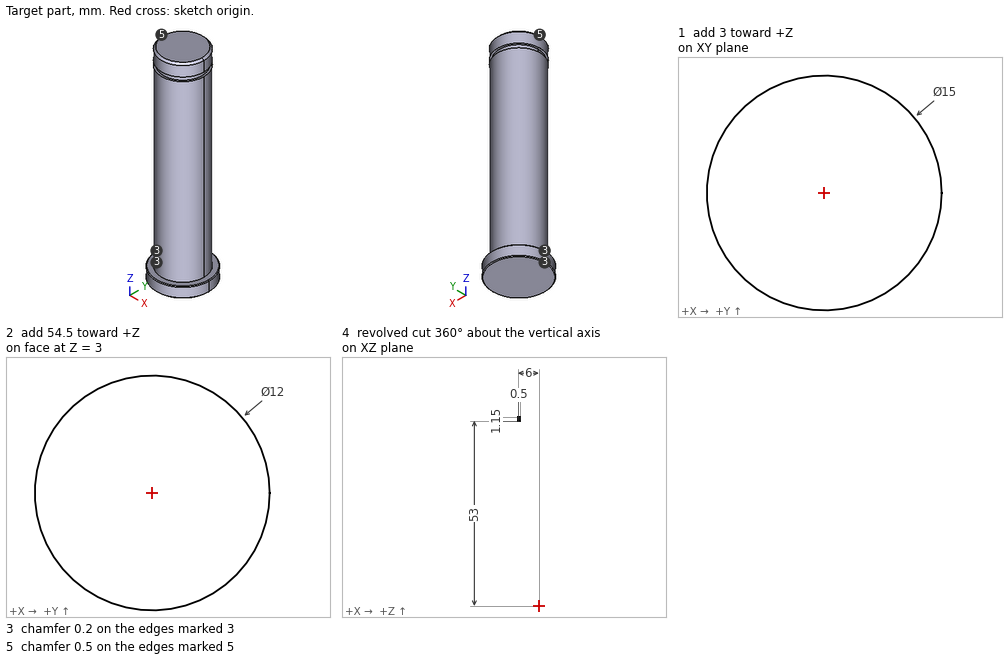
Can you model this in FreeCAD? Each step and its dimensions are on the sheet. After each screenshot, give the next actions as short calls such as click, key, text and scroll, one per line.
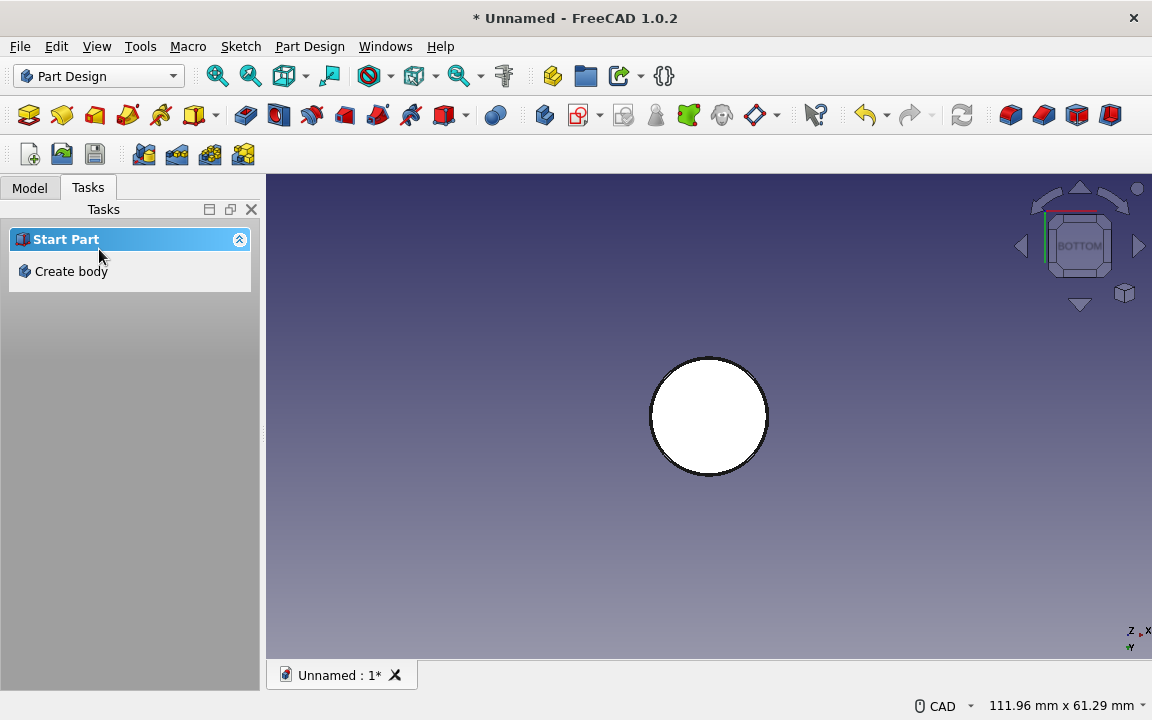
click(578, 116)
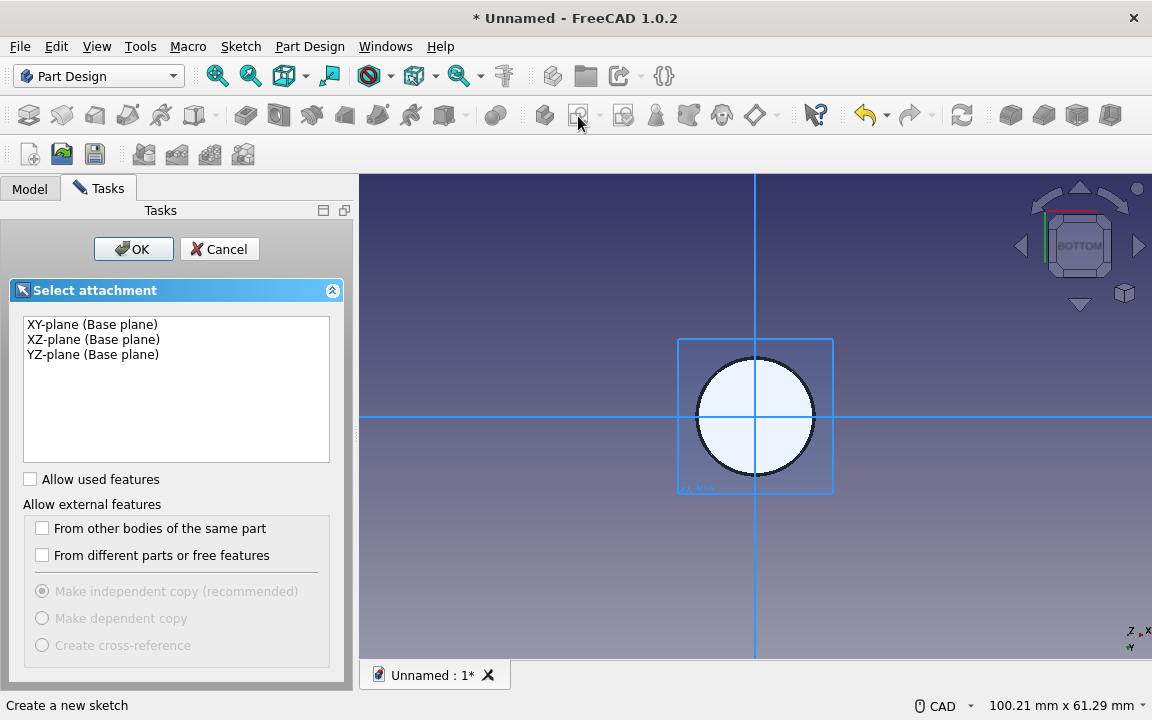
click(84, 340)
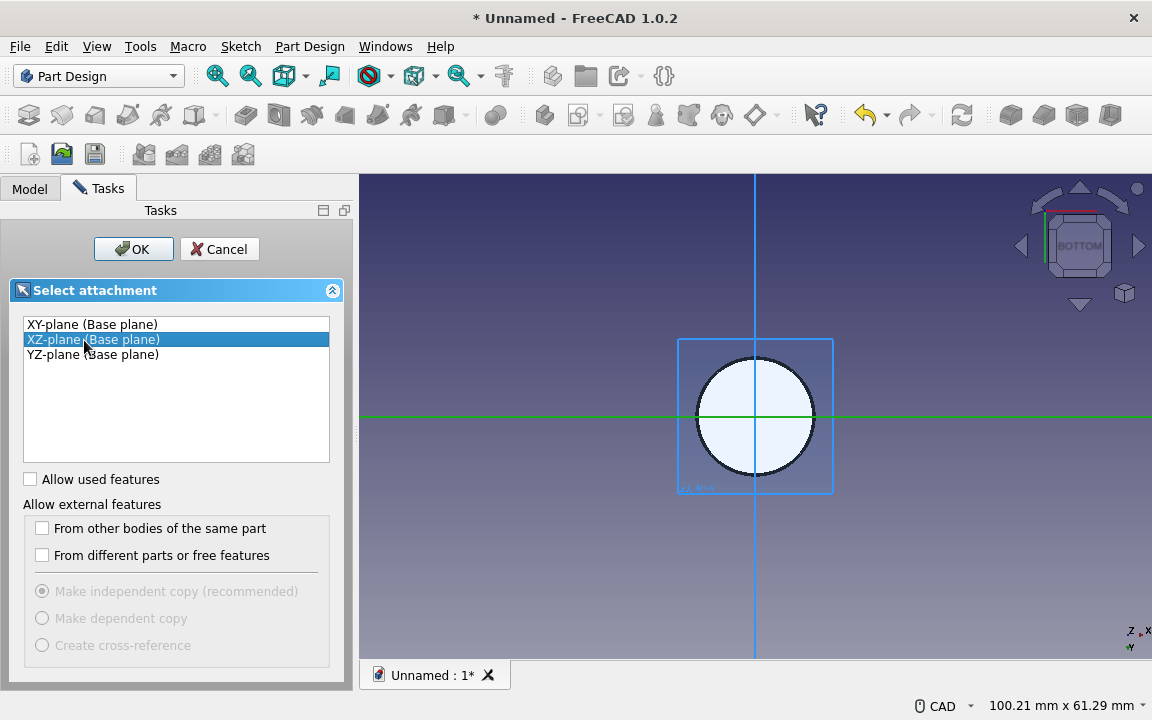
click(134, 249)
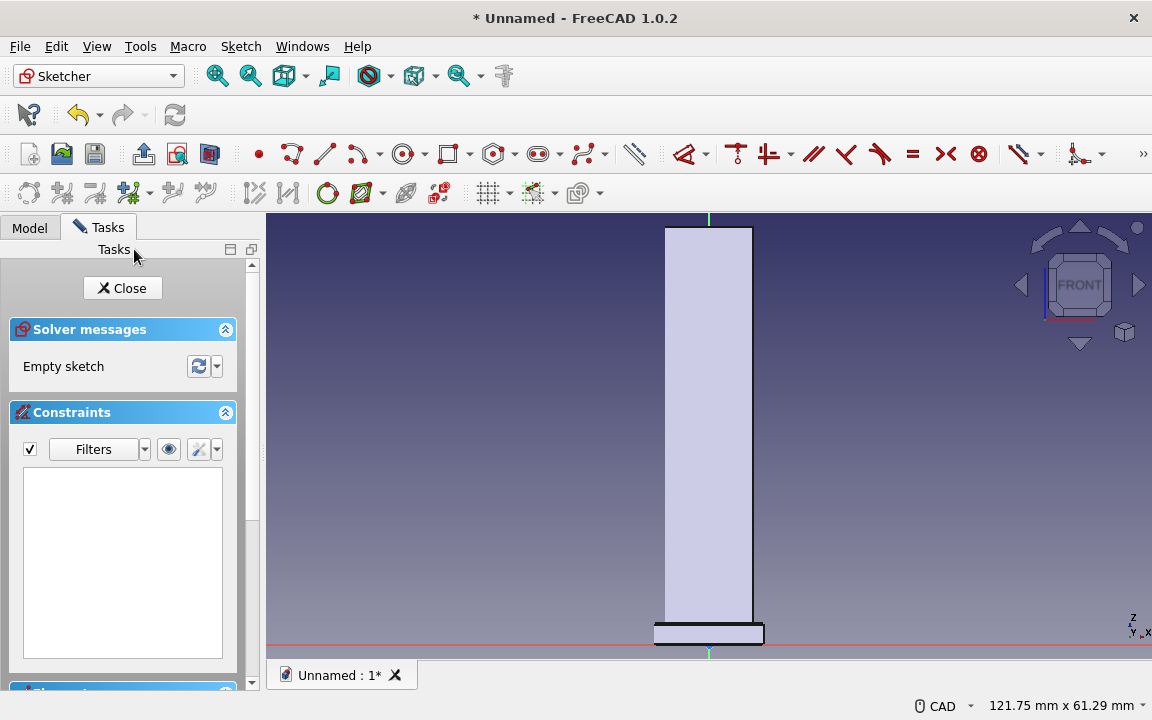
key(q)
key(s)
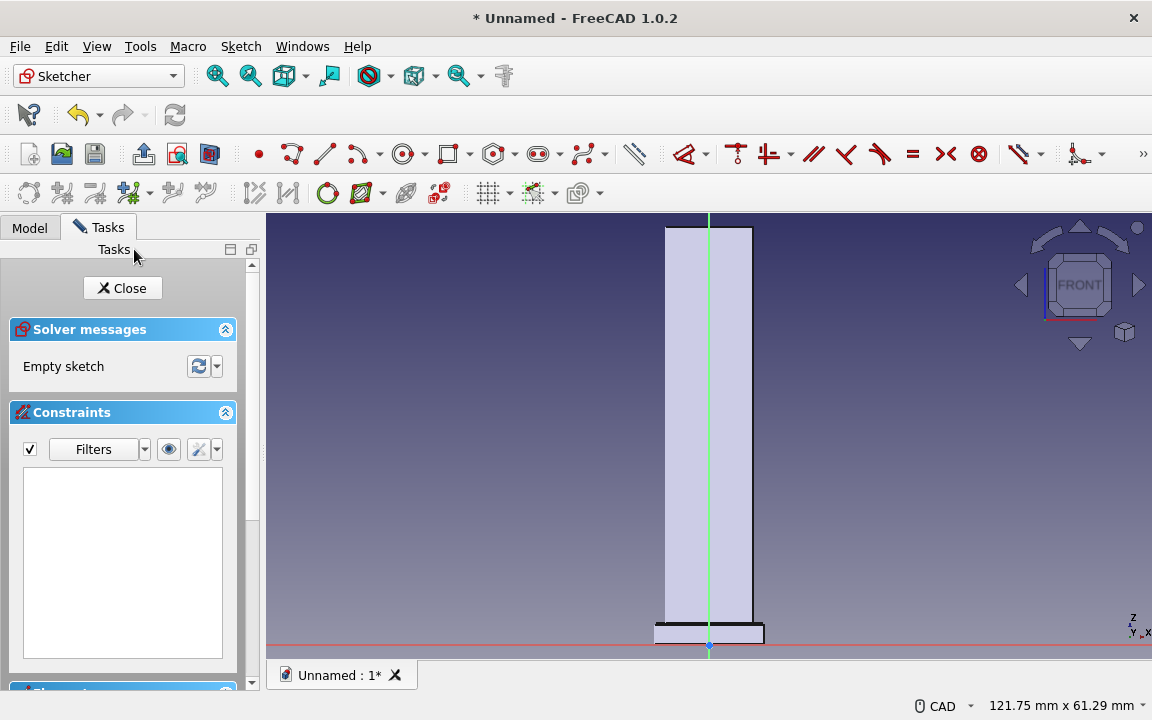
scroll(669, 246, up, 15)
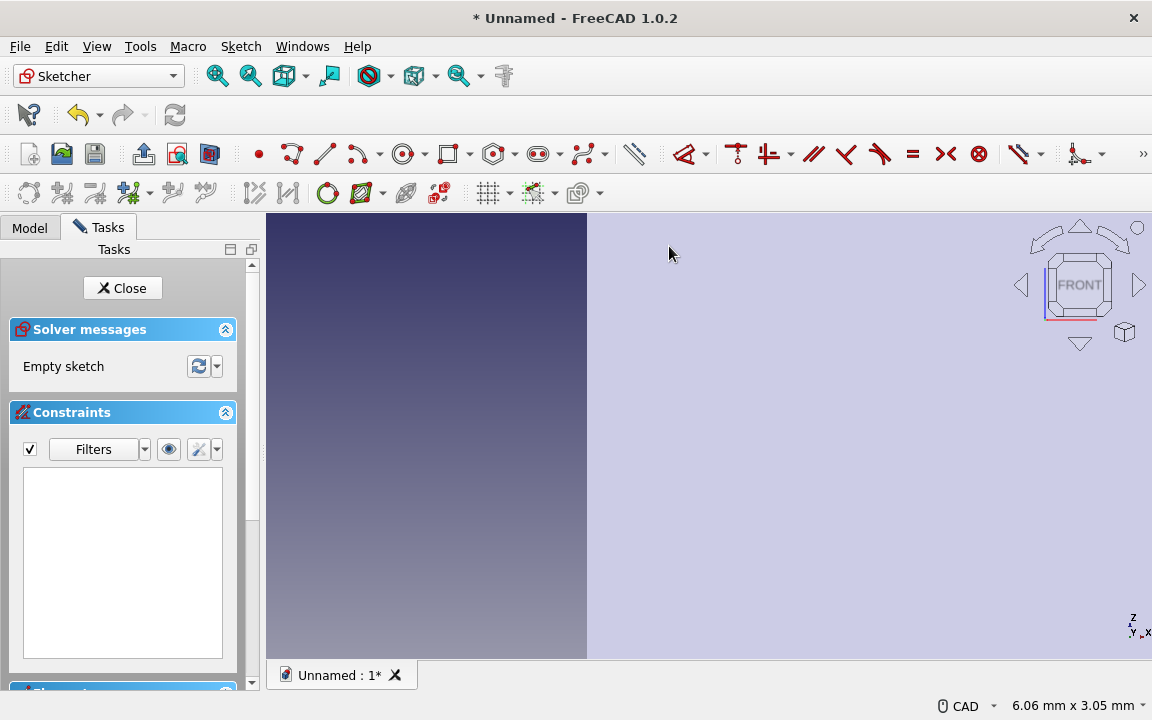
scroll(588, 425, up, 2)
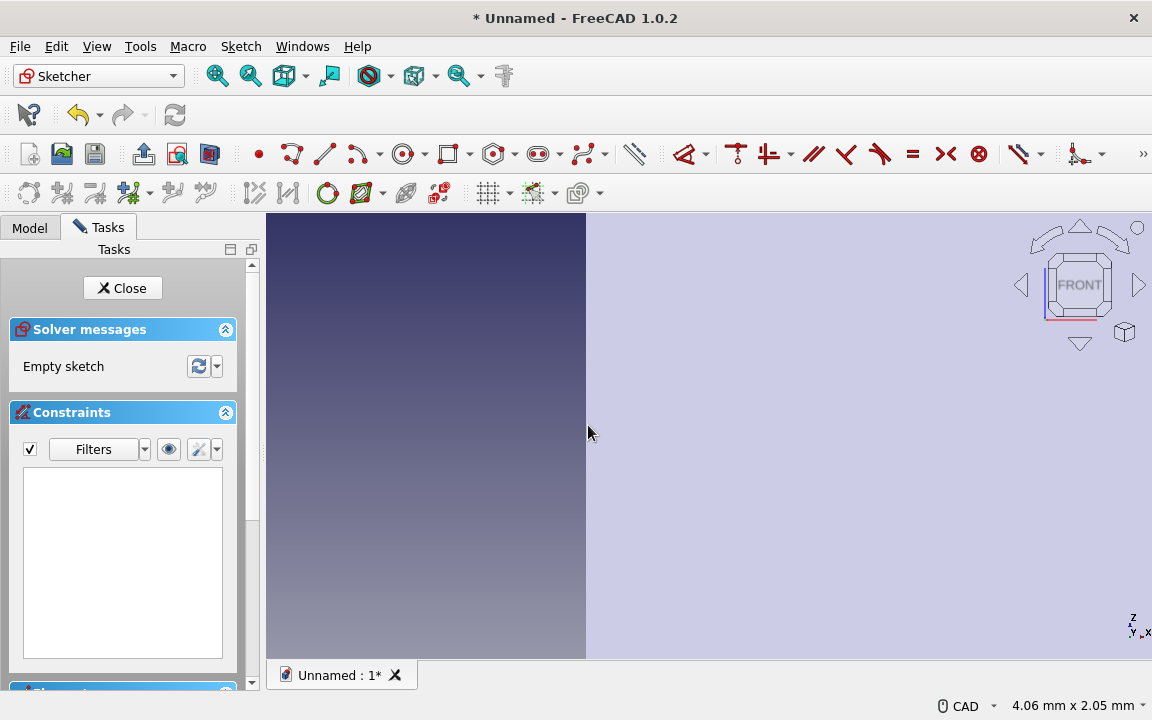
key(g)
key(r)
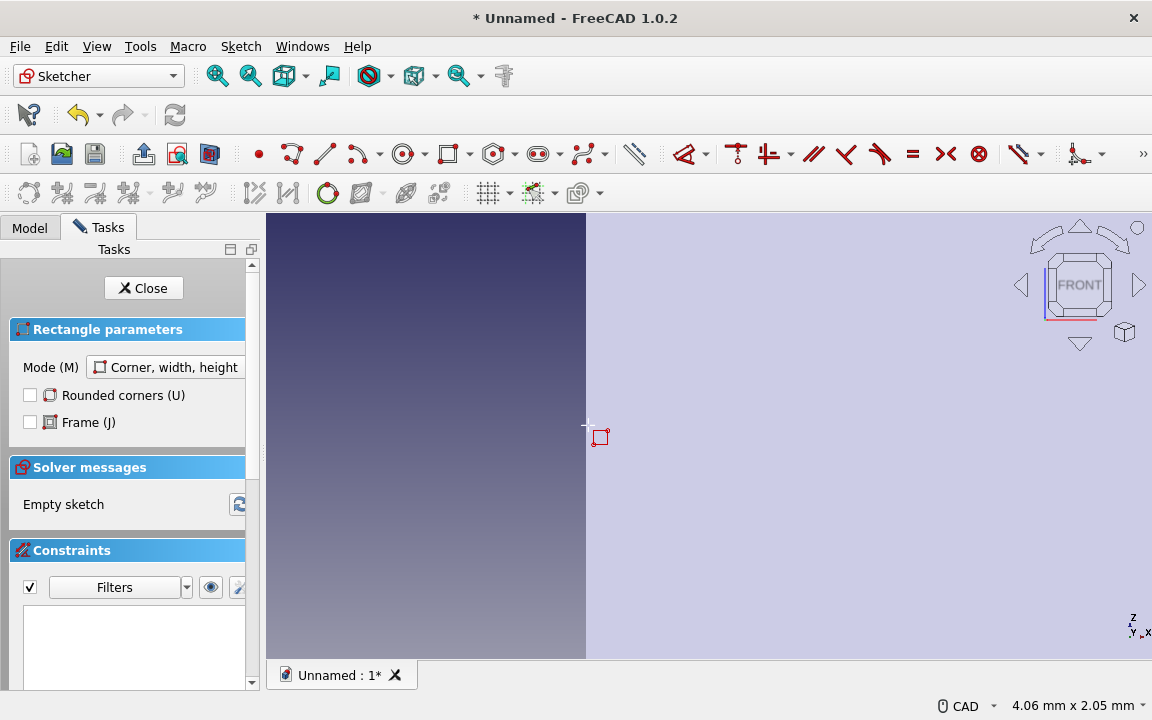
click(586, 310)
move(695, 561)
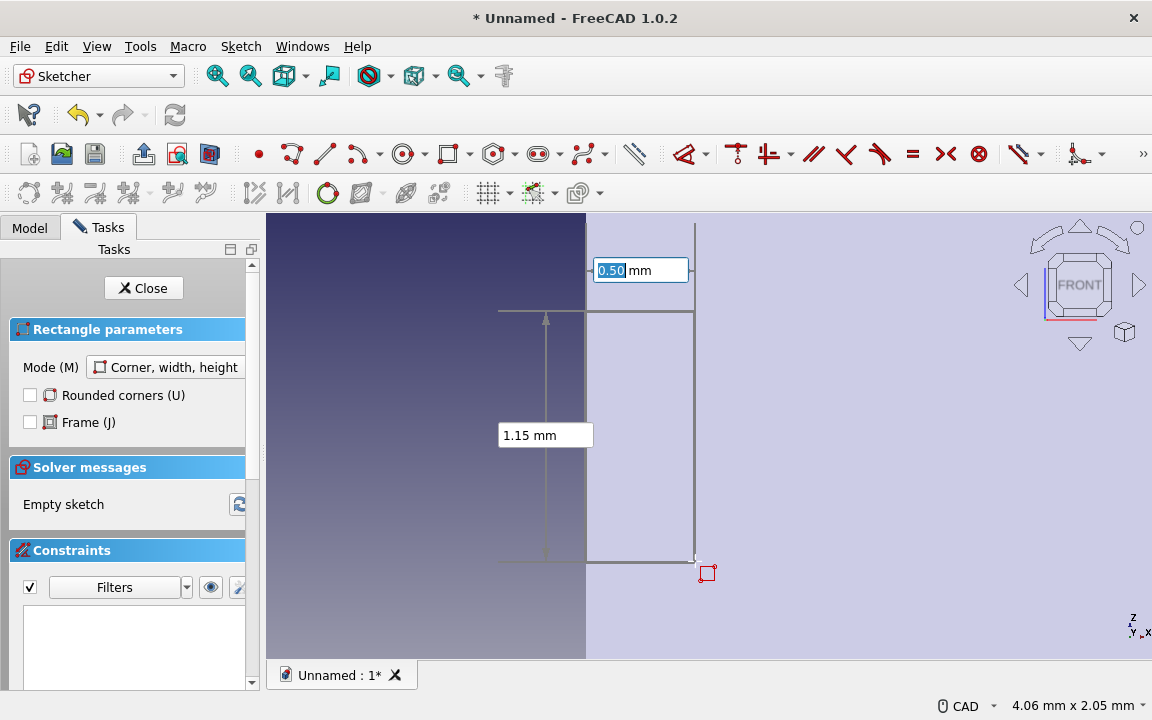
text(0.5)
key(Tab)
text(1.15)
key(Return)
key(Escape)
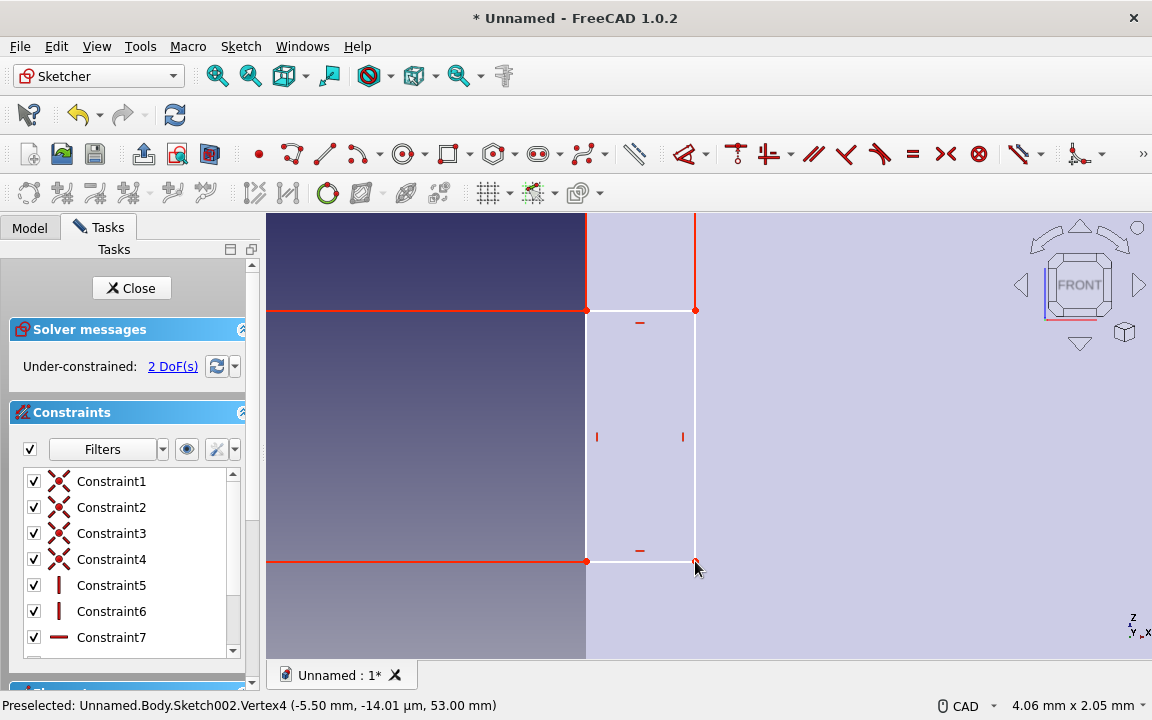
click(586, 311)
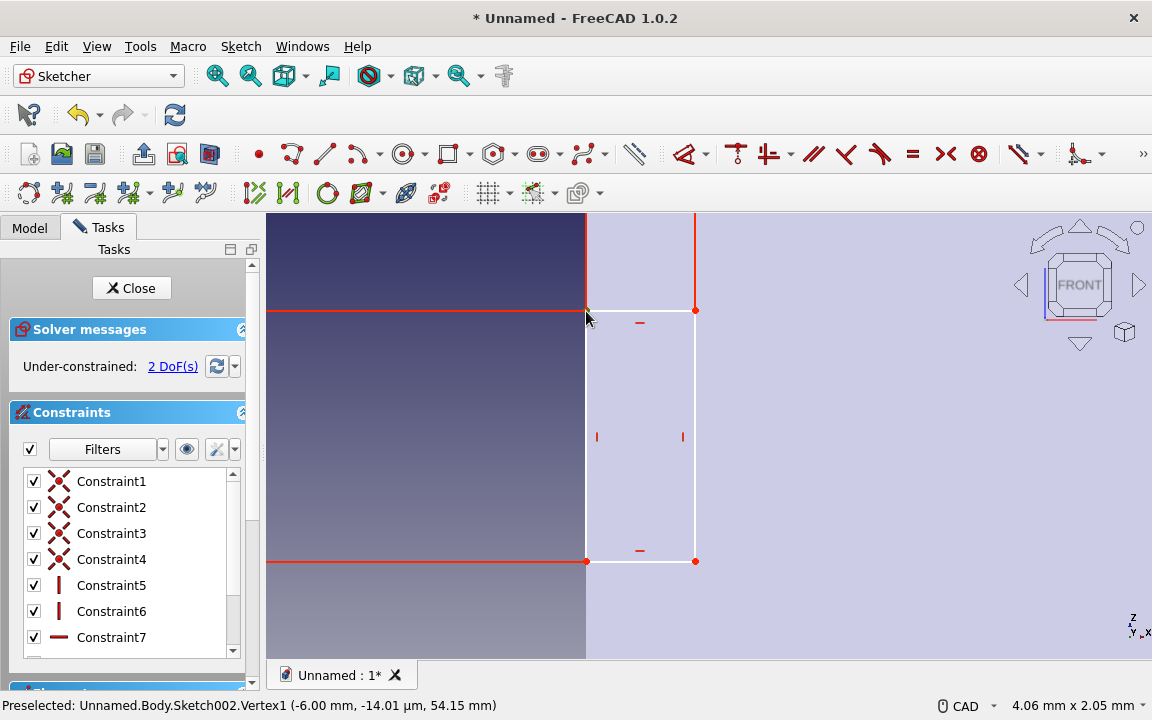
key(l)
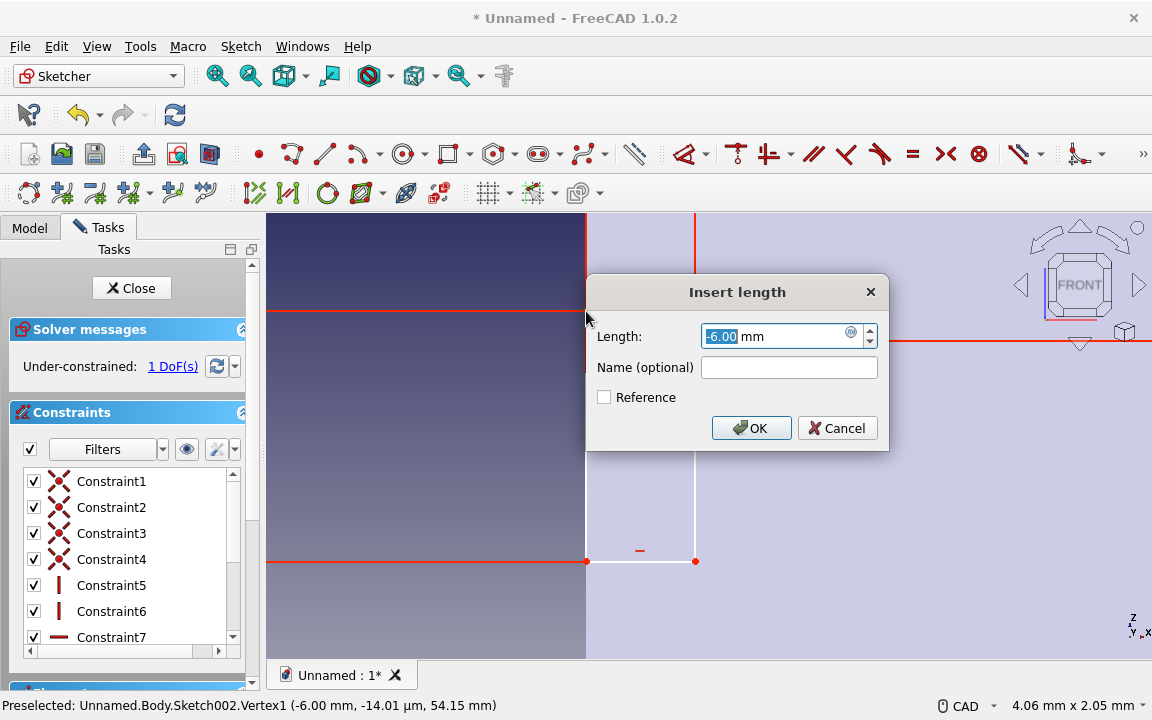
text(-6)
key(Return)